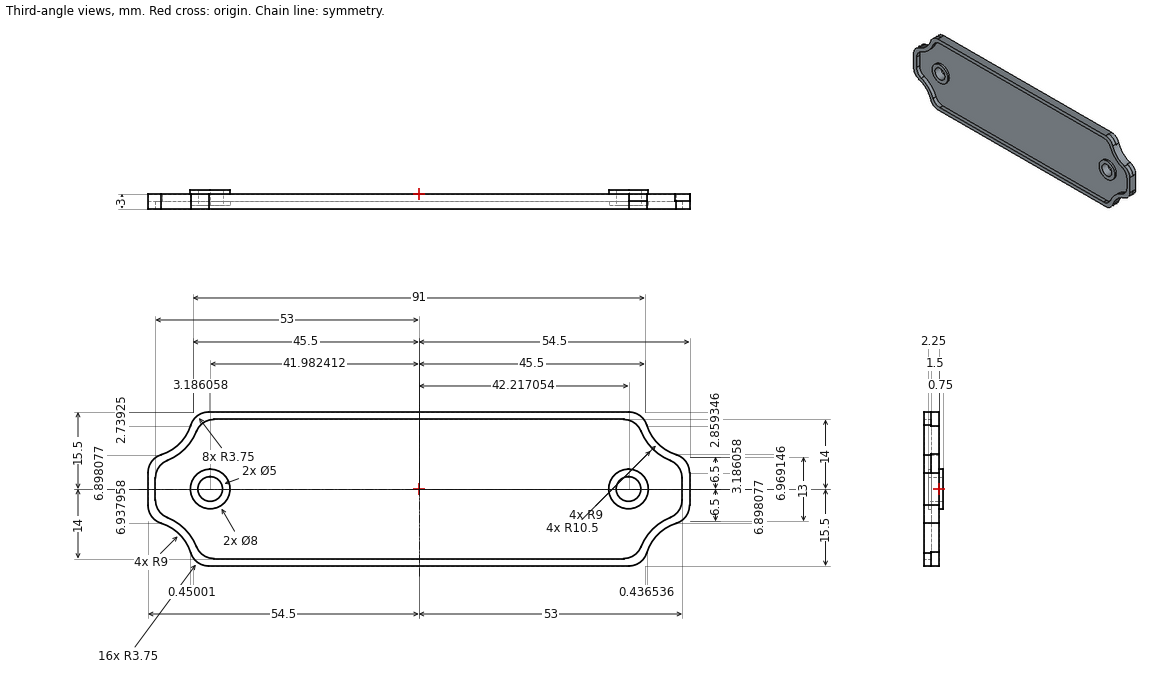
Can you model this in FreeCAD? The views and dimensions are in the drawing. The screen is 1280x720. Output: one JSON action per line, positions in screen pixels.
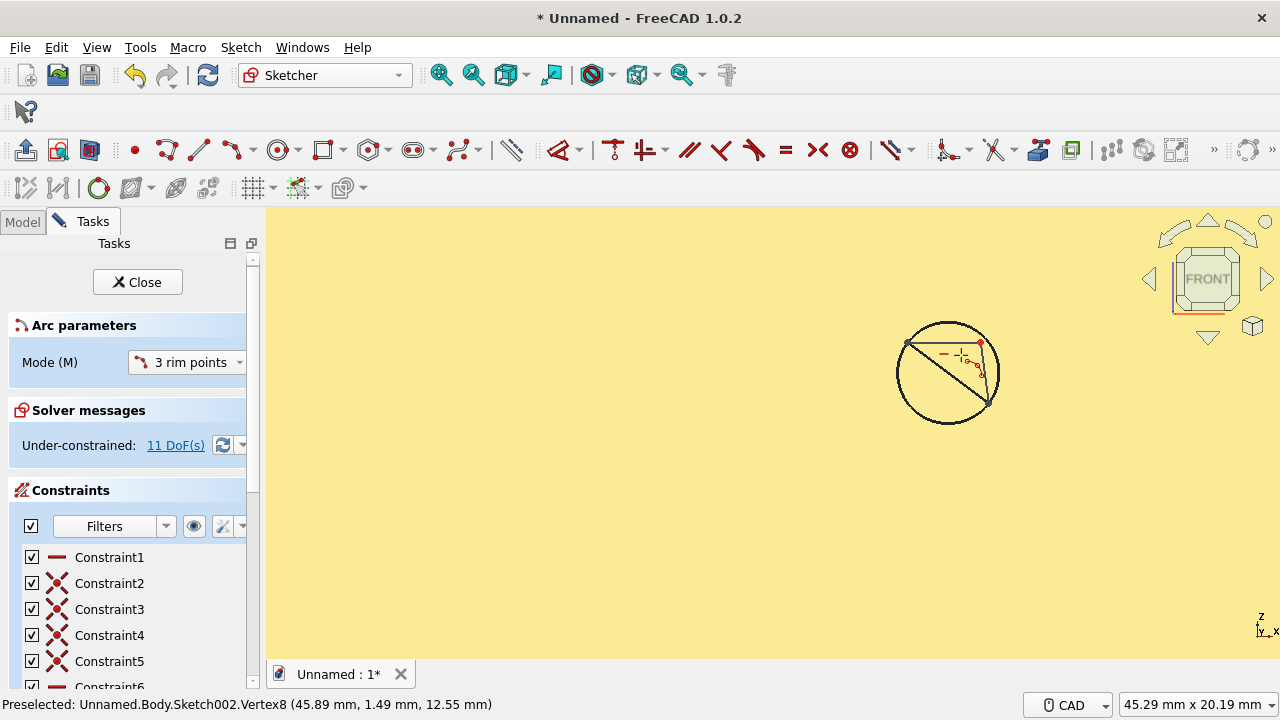
{"action": "left_click", "coordinate": [961, 355]}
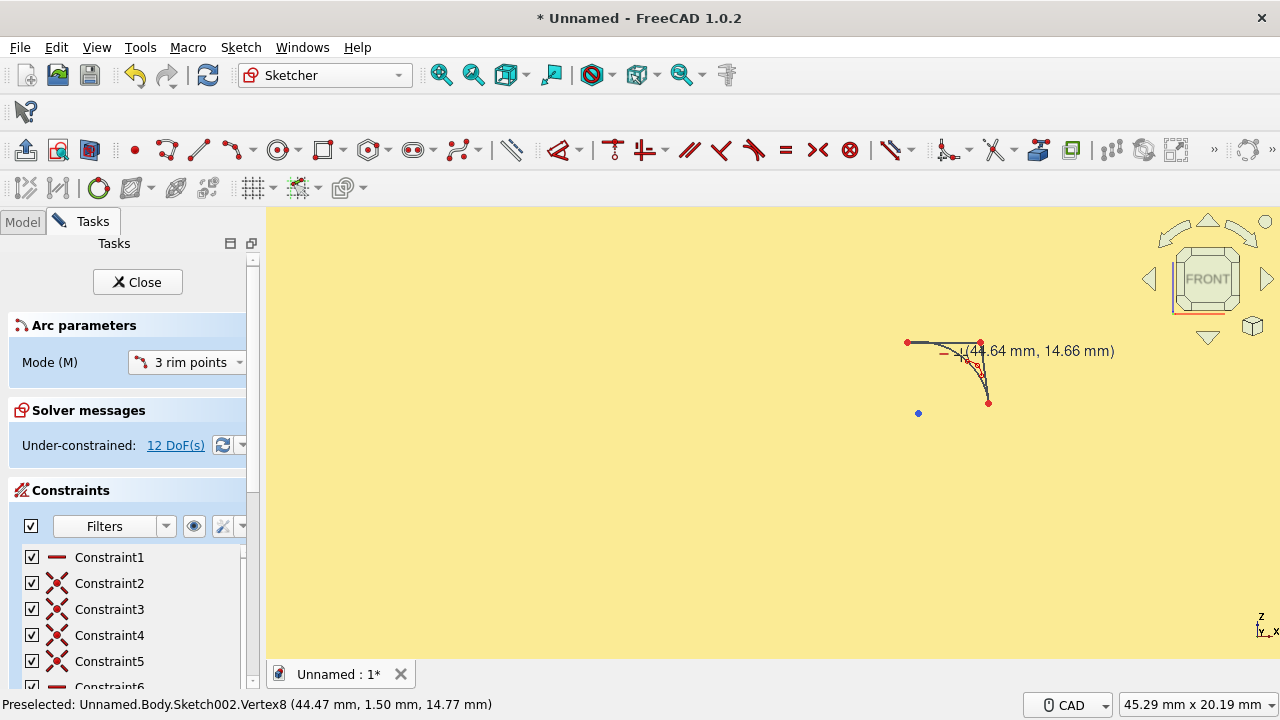
{"action": "left_click", "coordinate": [168, 150]}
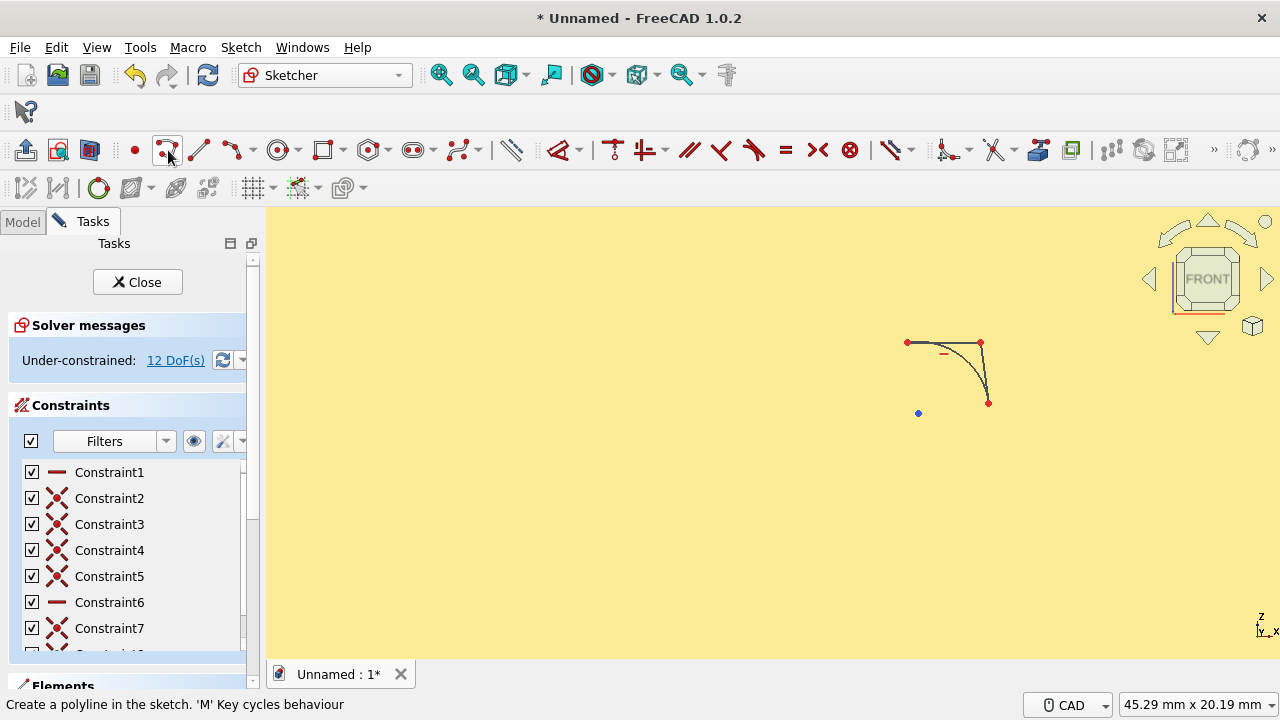
{"action": "scroll", "coordinate": [948, 351], "scroll_direction": "down", "scroll_amount": 7}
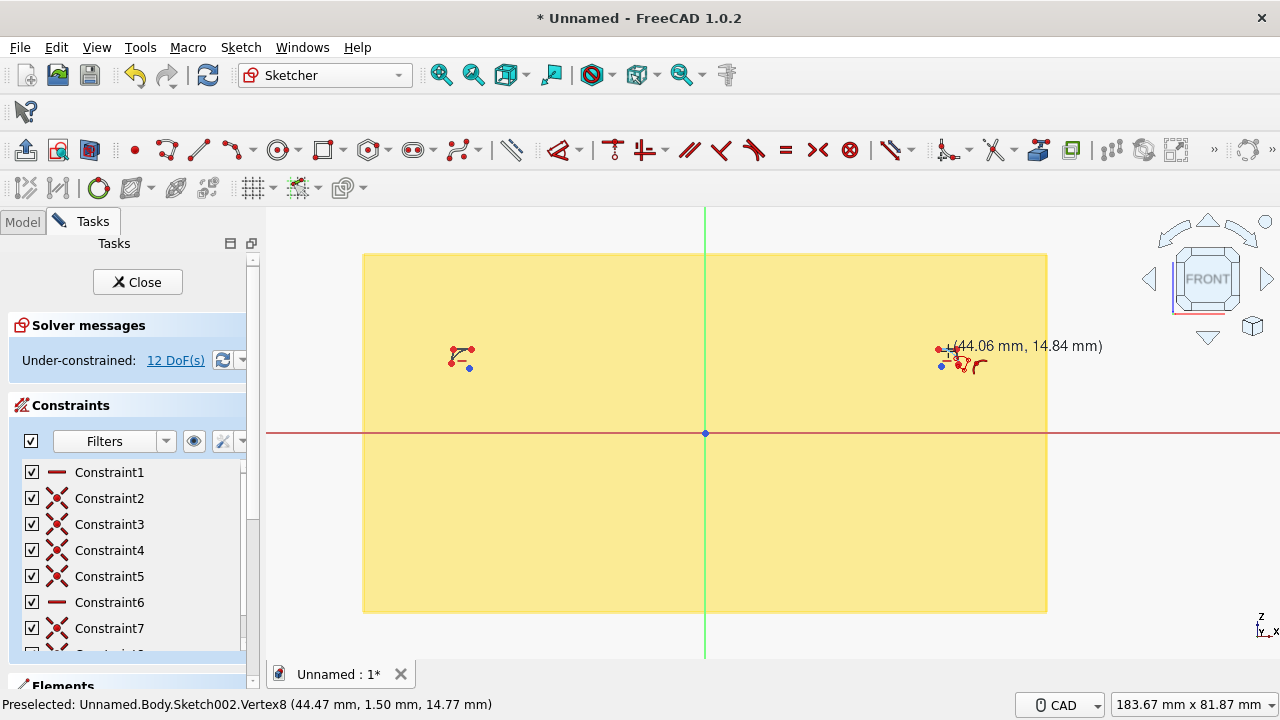
{"action": "left_click", "coordinate": [1006, 415]}
{"action": "left_click", "coordinate": [1006, 398]}
{"action": "left_click", "coordinate": [990, 395]}
{"action": "right_click", "coordinate": [990, 395]}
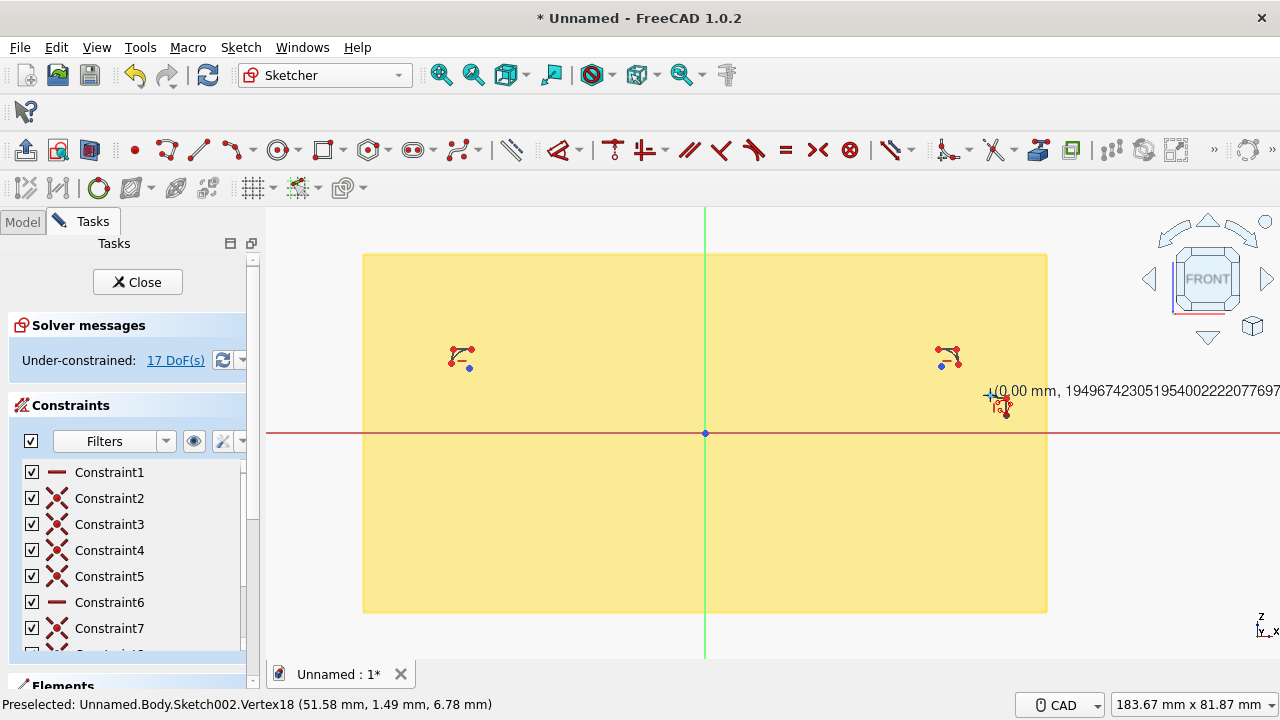
{"action": "left_click", "coordinate": [232, 150]}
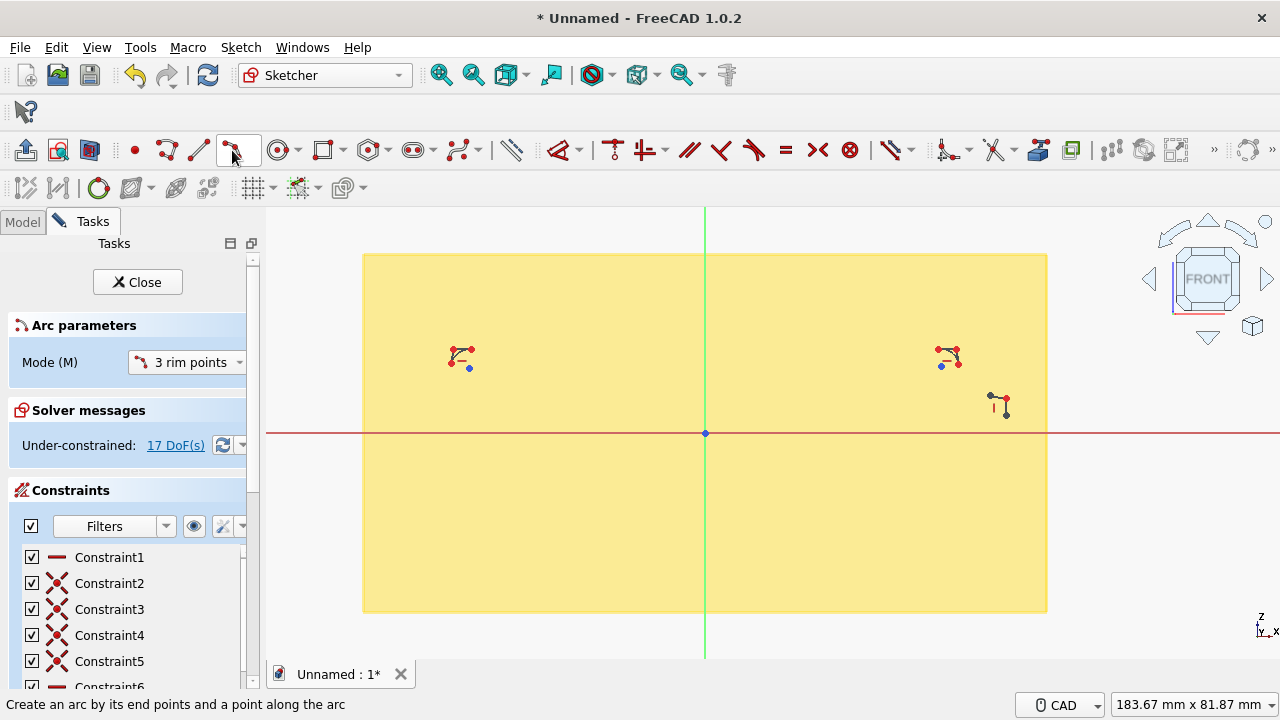
{"action": "scroll", "coordinate": [990, 395], "scroll_direction": "up", "scroll_amount": 4}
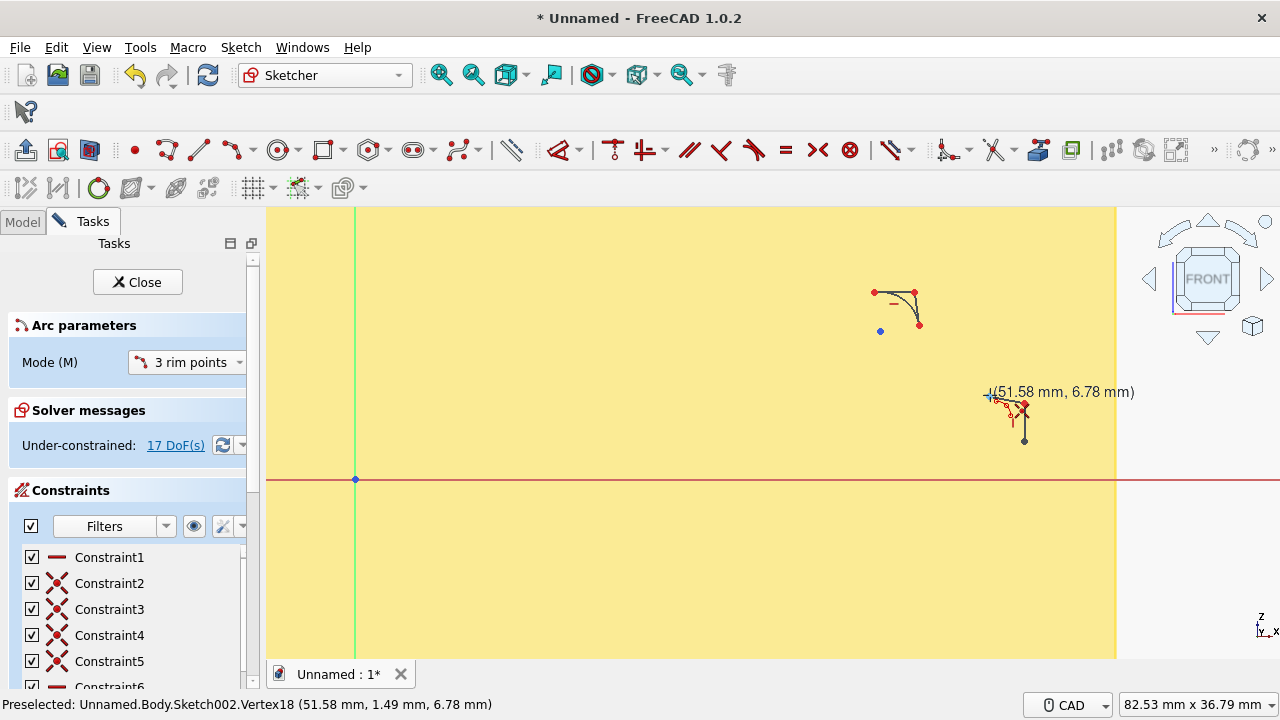
{"action": "left_click", "coordinate": [989, 397]}
{"action": "left_click", "coordinate": [1025, 441]}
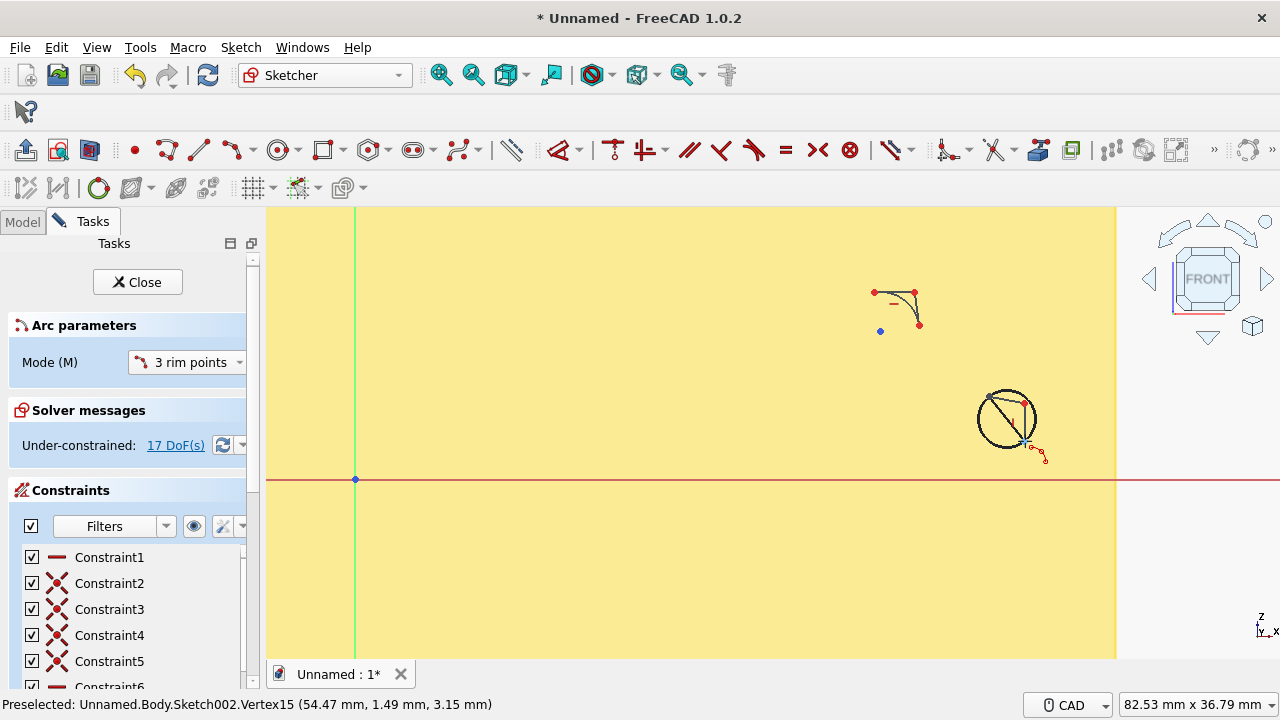
{"action": "scroll", "coordinate": [1015, 411], "scroll_direction": "up", "scroll_amount": 3}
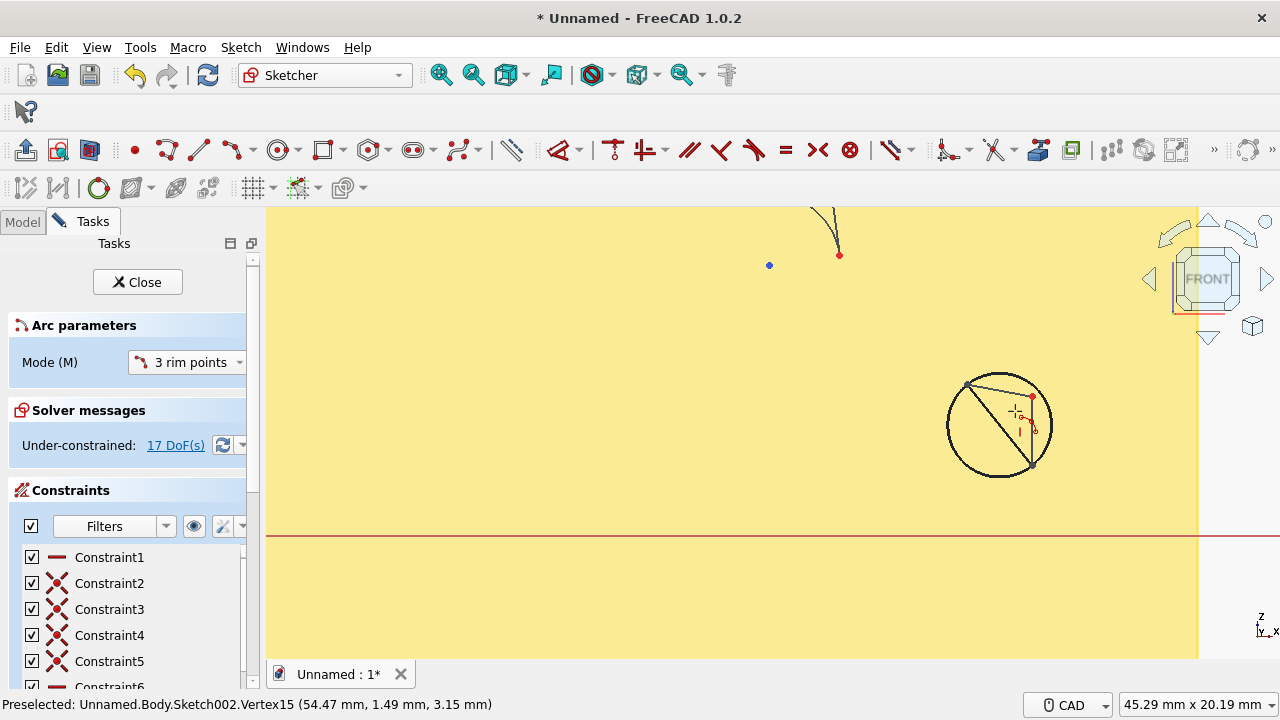
{"action": "left_click", "coordinate": [1014, 410]}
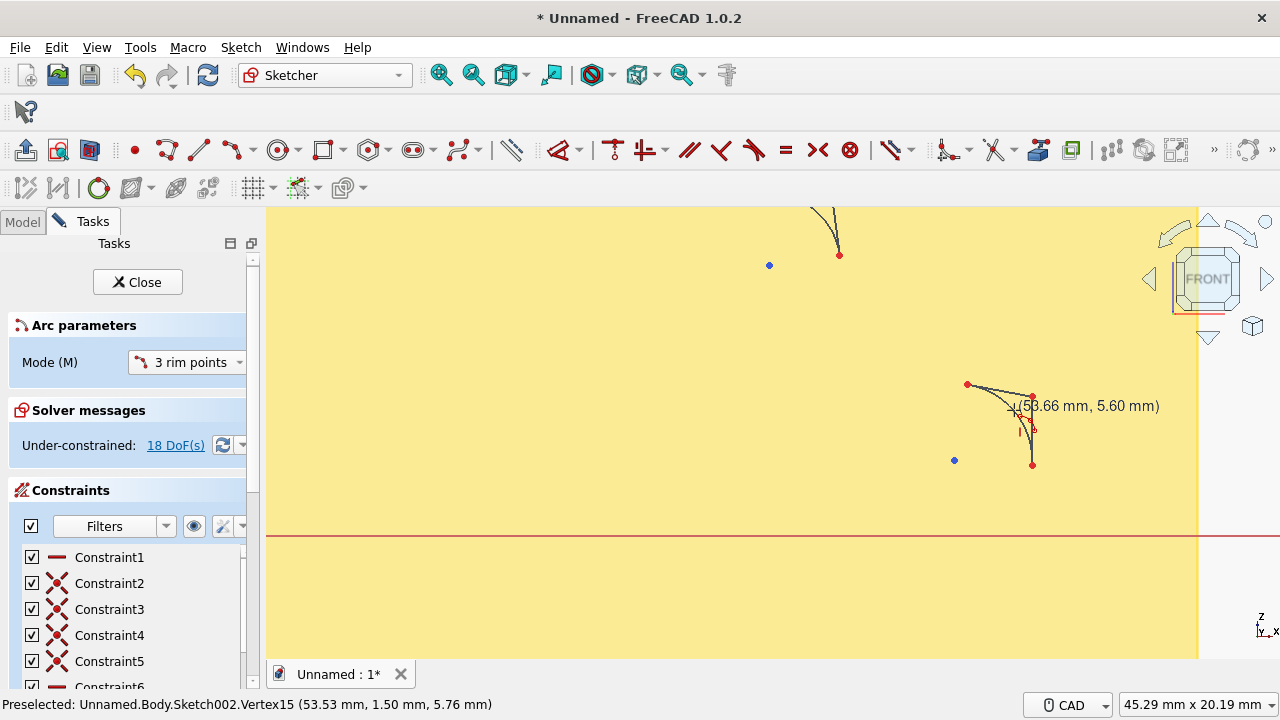
{"action": "left_click", "coordinate": [168, 150]}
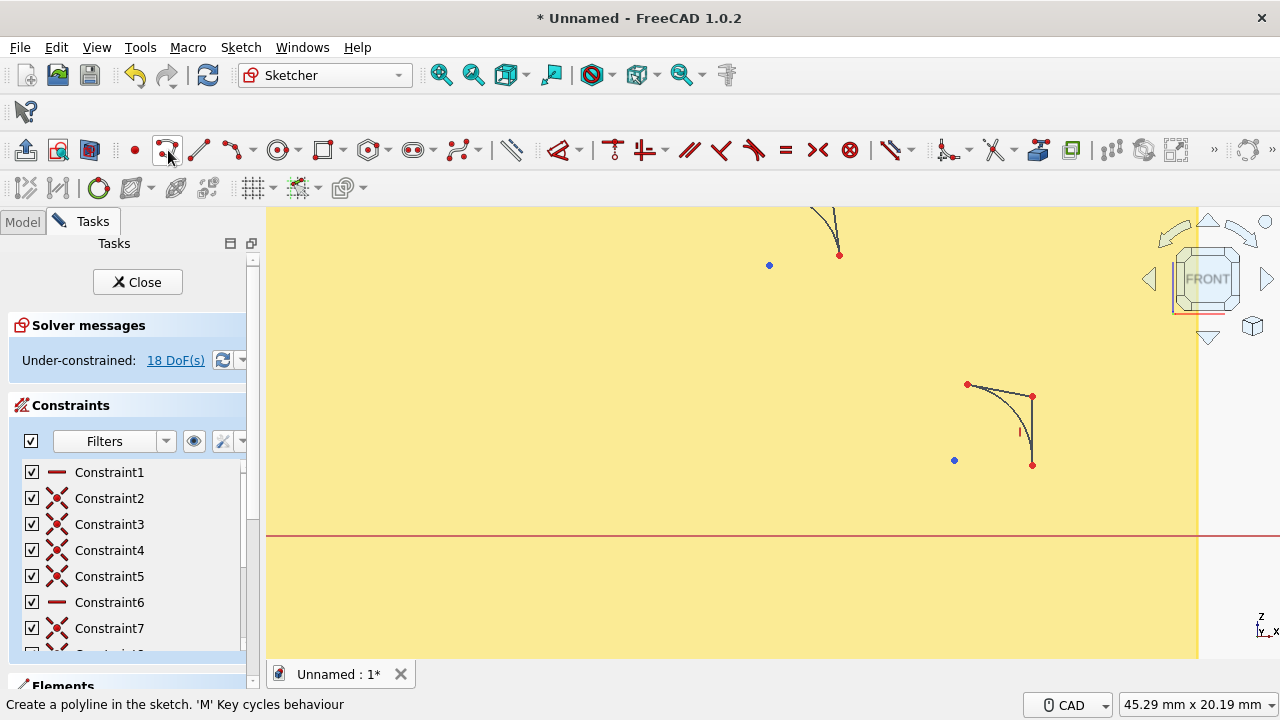
{"action": "scroll", "coordinate": [996, 399], "scroll_direction": "down", "scroll_amount": 7}